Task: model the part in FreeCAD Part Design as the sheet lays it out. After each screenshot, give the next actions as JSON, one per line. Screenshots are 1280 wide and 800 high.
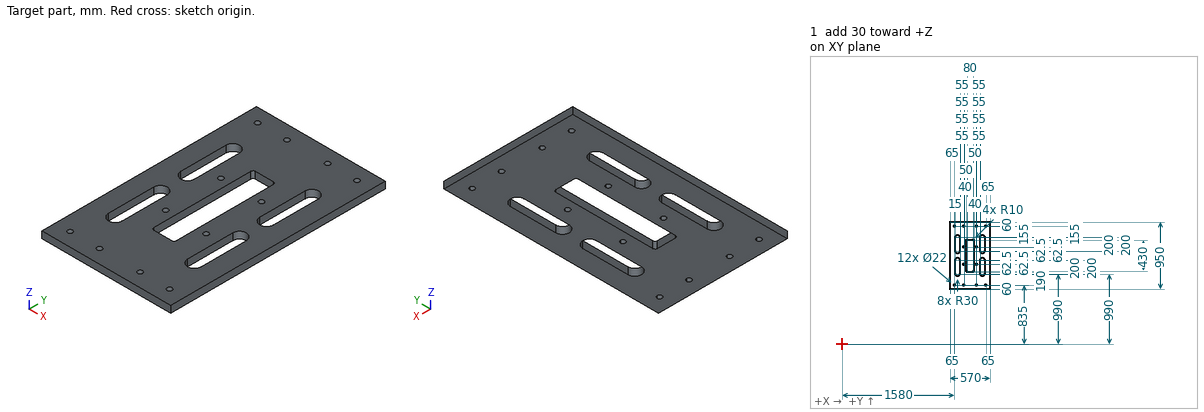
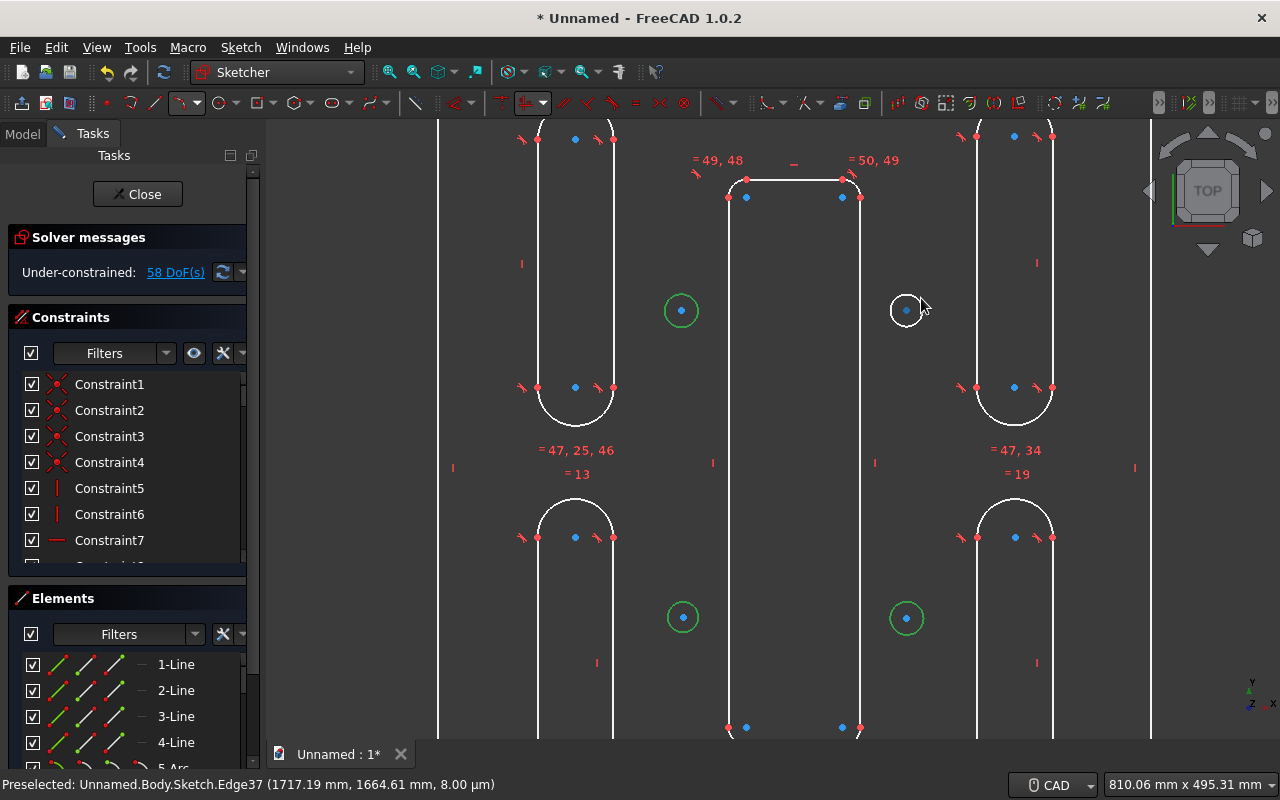
{"action": "left_click", "coordinate": [918, 299]}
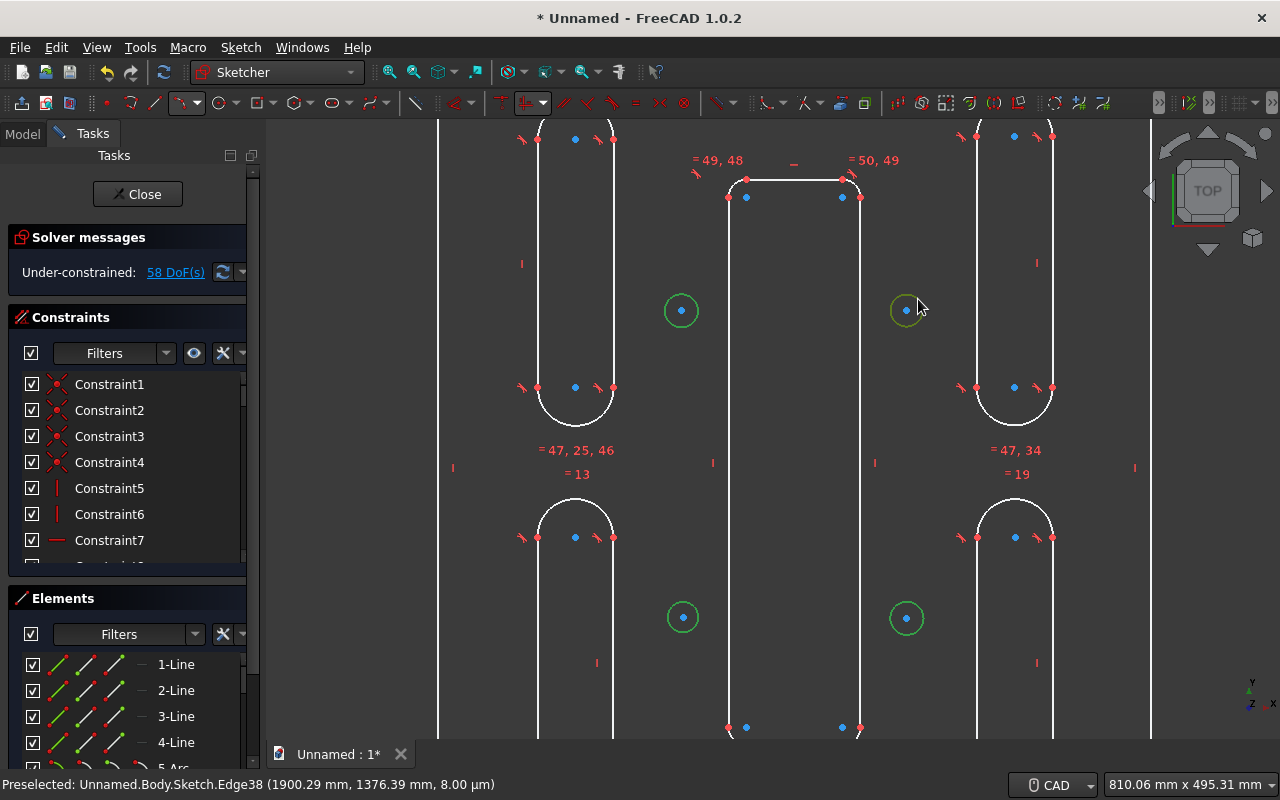
{"action": "scroll", "coordinate": [921, 298], "scroll_direction": "down", "scroll_amount": 8}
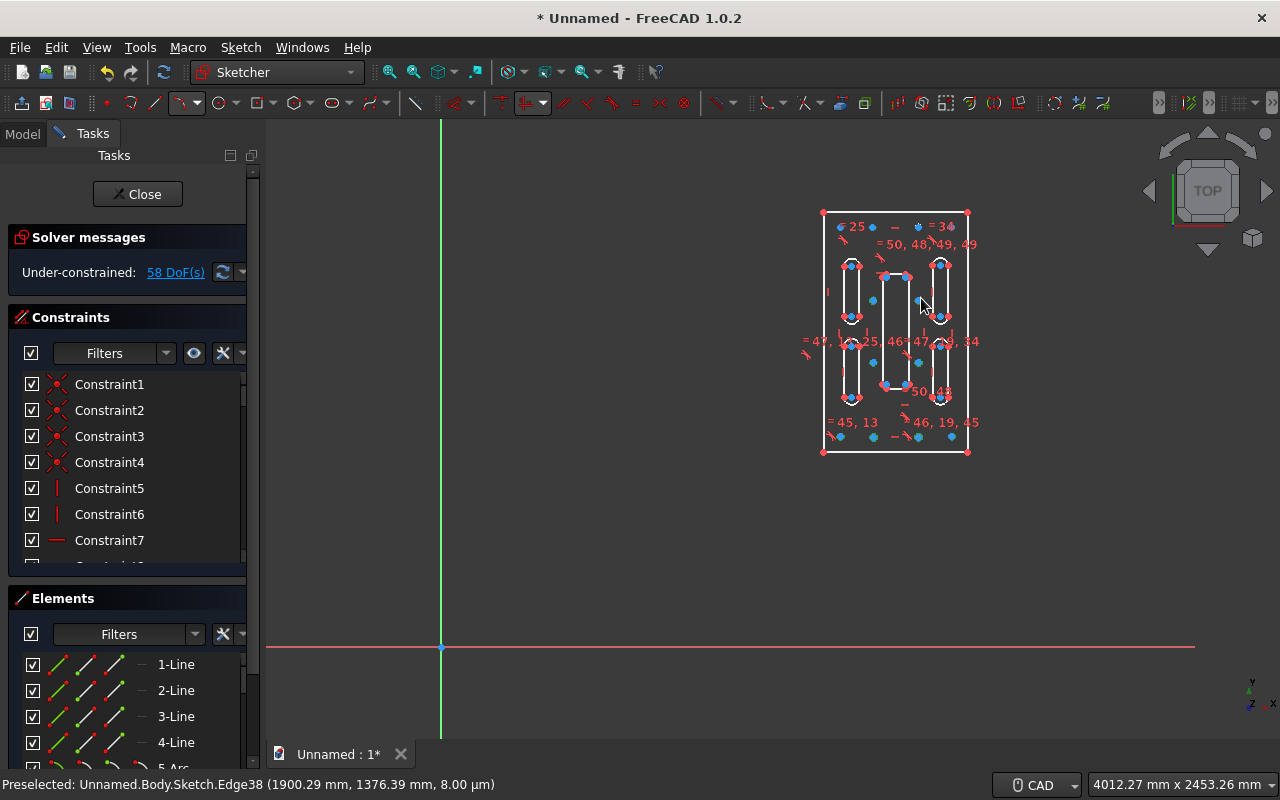
{"action": "scroll", "coordinate": [920, 225], "scroll_direction": "up", "scroll_amount": 9}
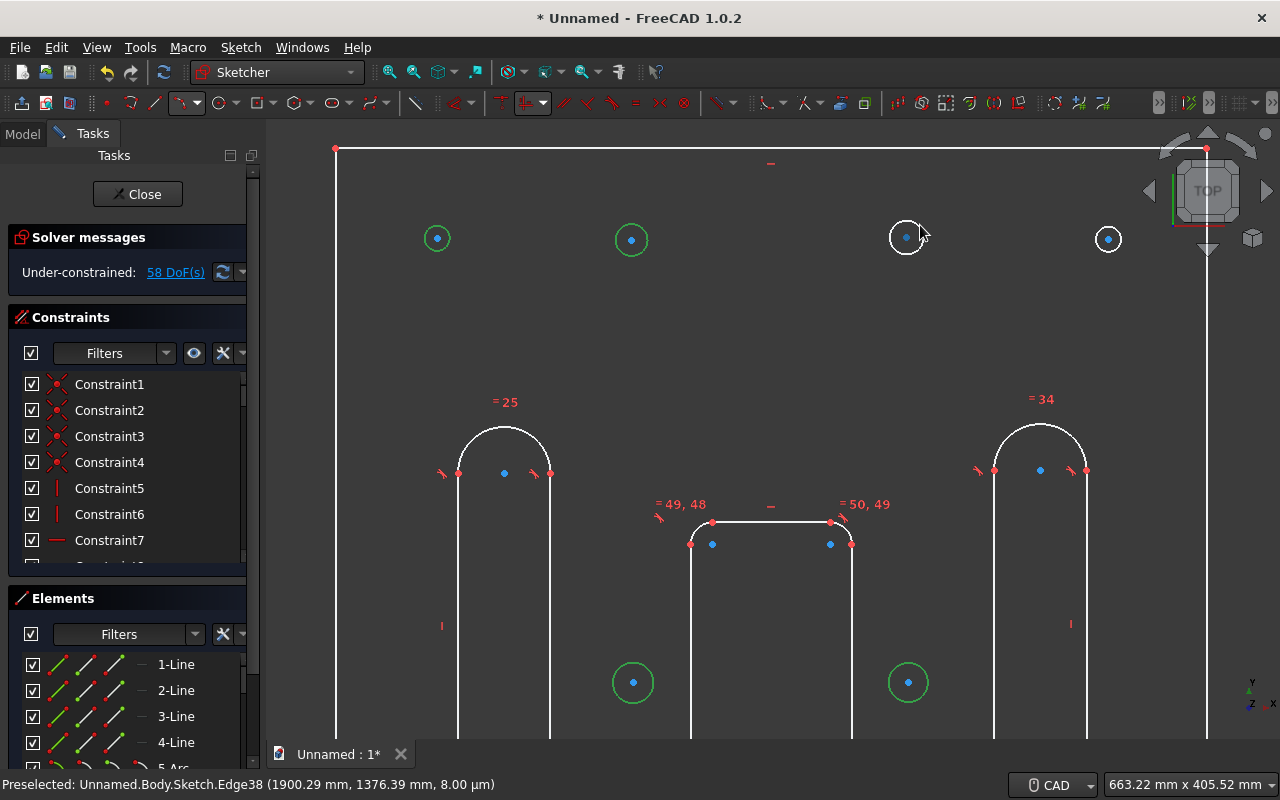
{"action": "left_click", "coordinate": [919, 226]}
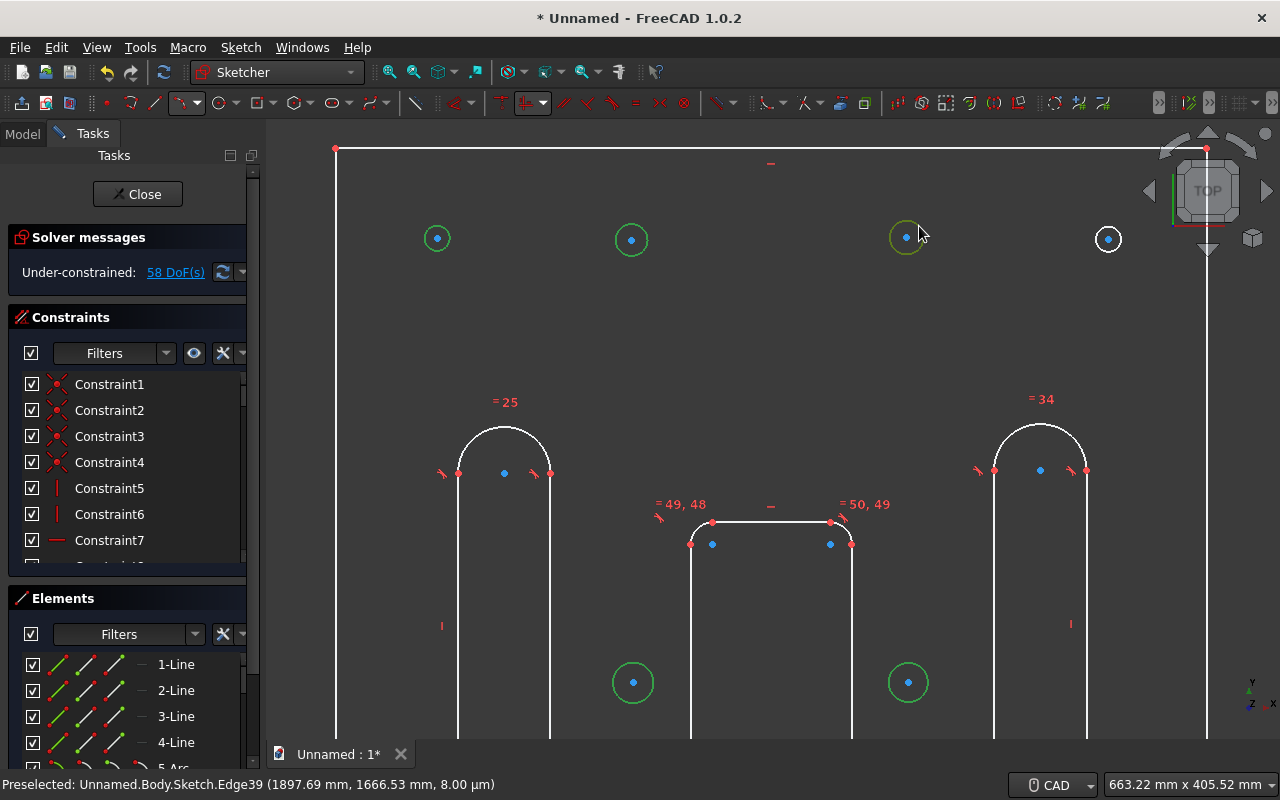
{"action": "left_click", "coordinate": [1100, 230]}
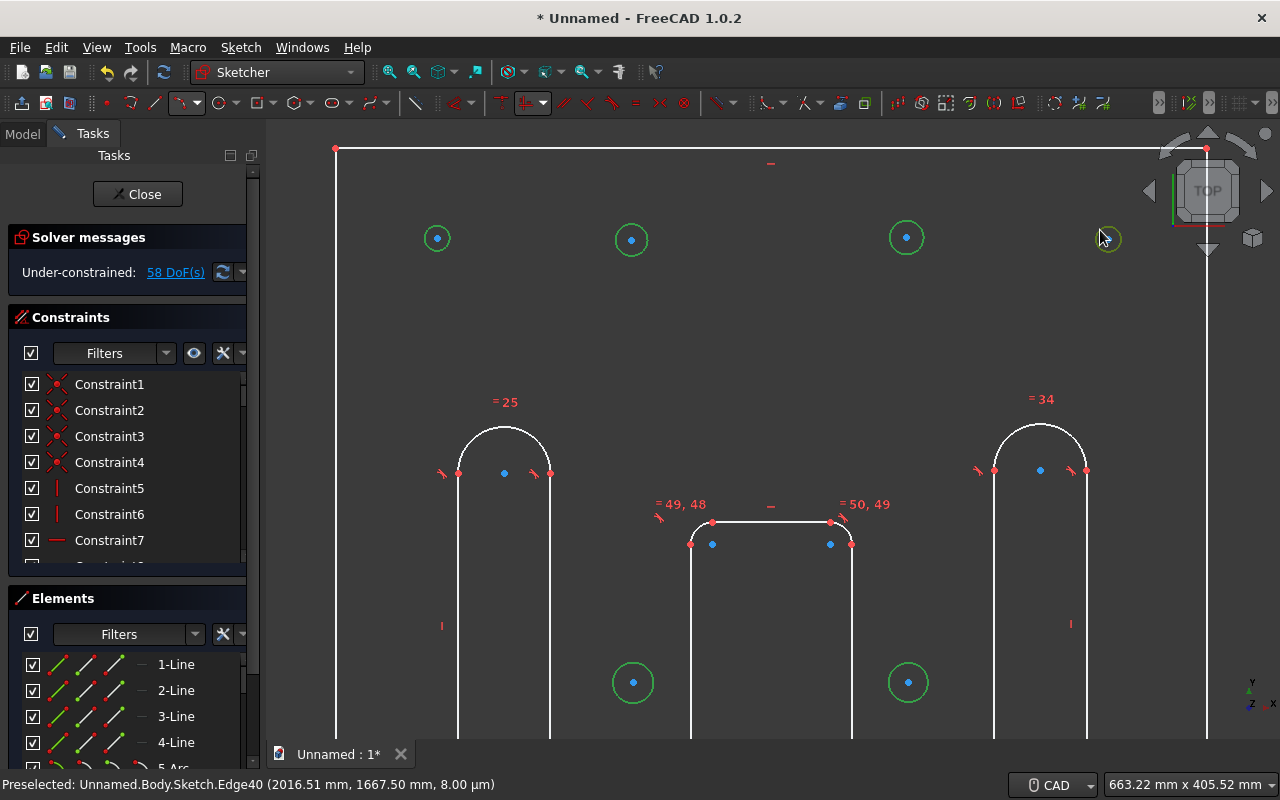
{"action": "left_click", "coordinate": [636, 104]}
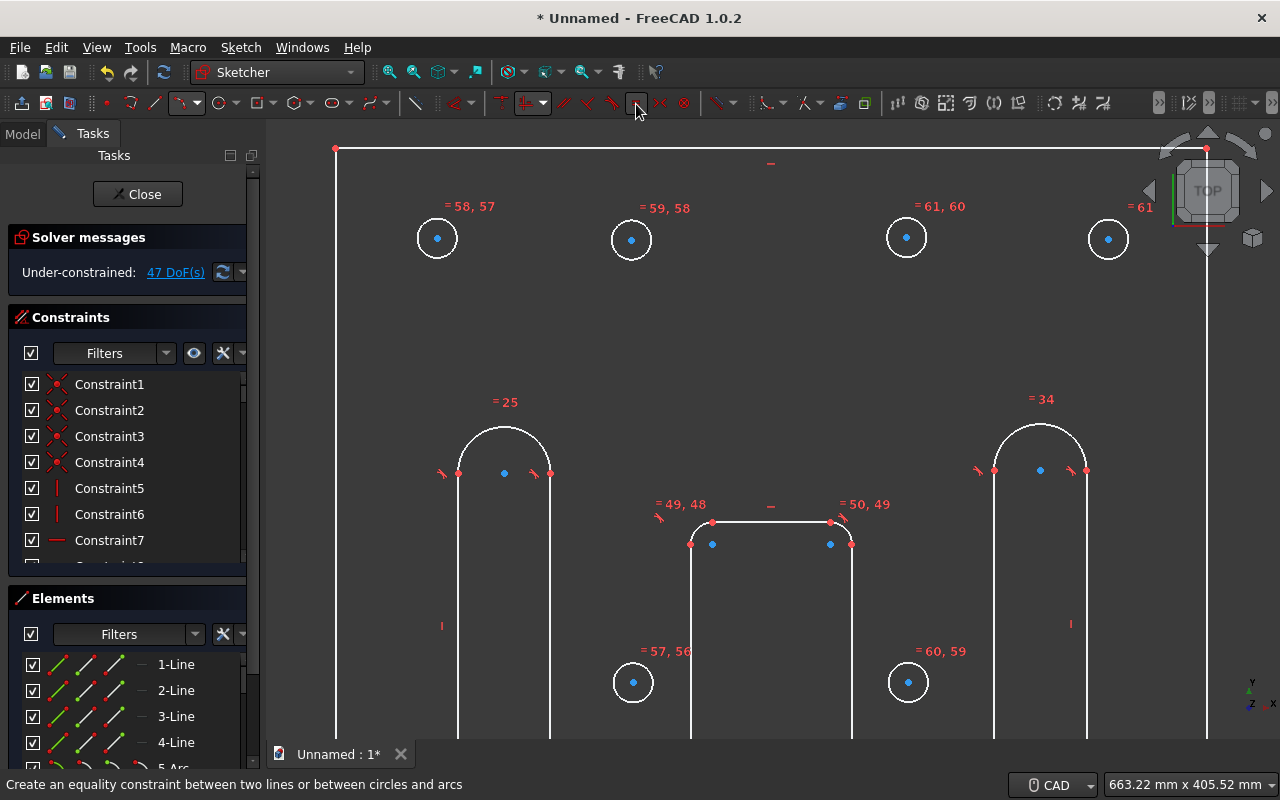
{"action": "scroll", "coordinate": [920, 225], "scroll_direction": "down", "scroll_amount": 9}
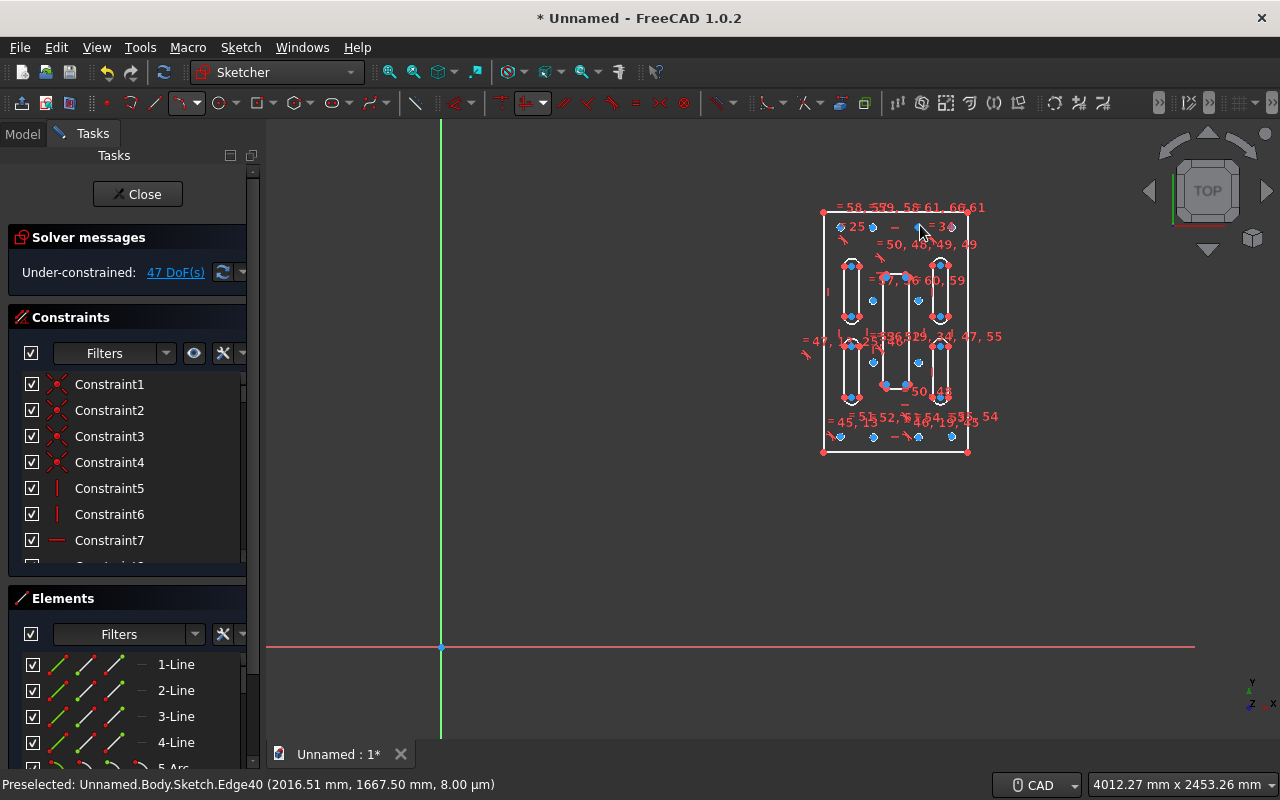
{"action": "left_click", "coordinate": [841, 437]}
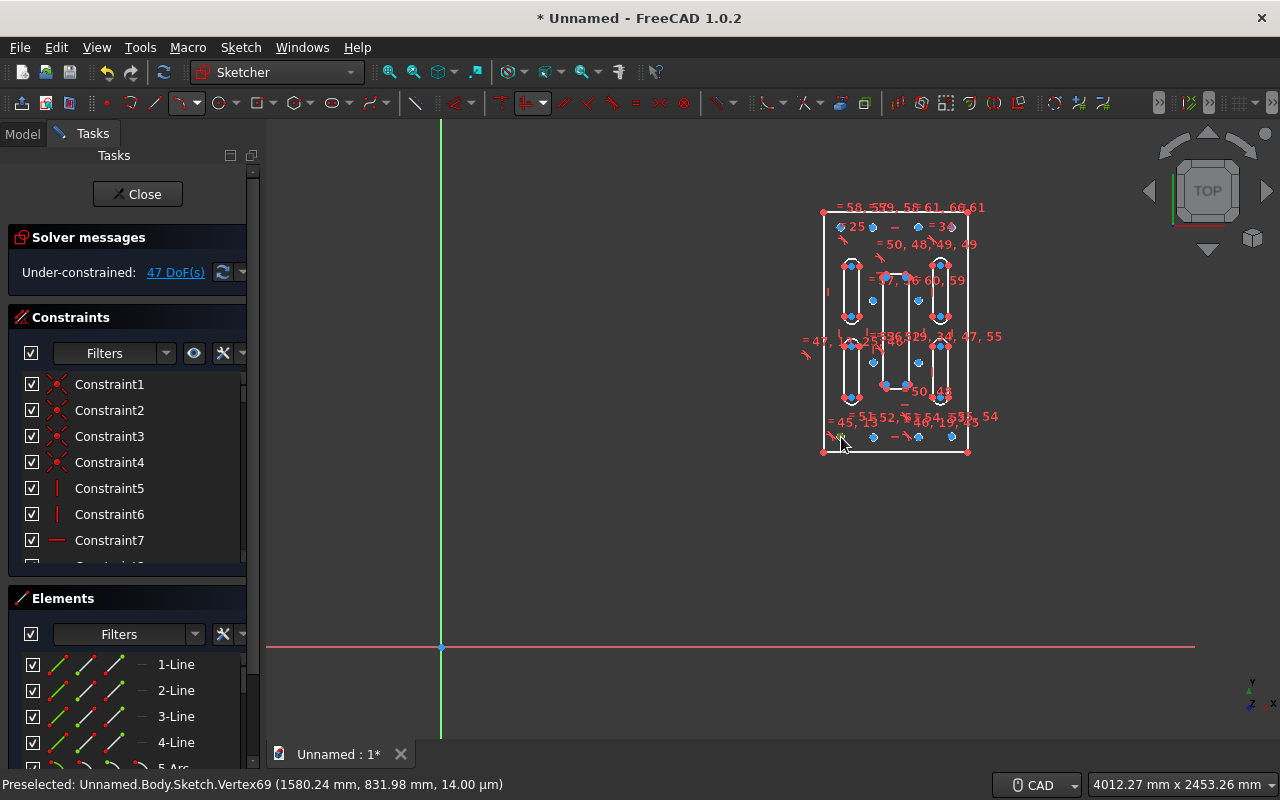
{"action": "left_click", "coordinate": [874, 437]}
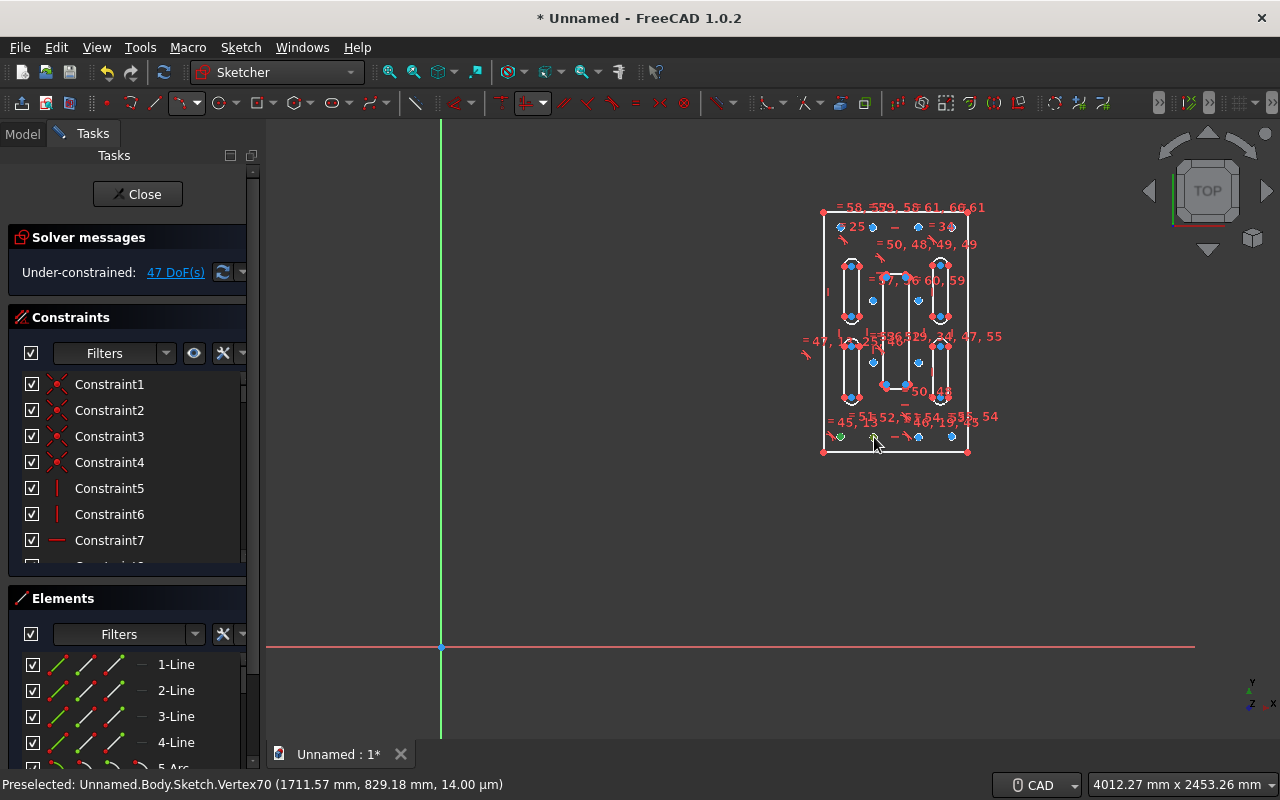
{"action": "key", "text": "h"}